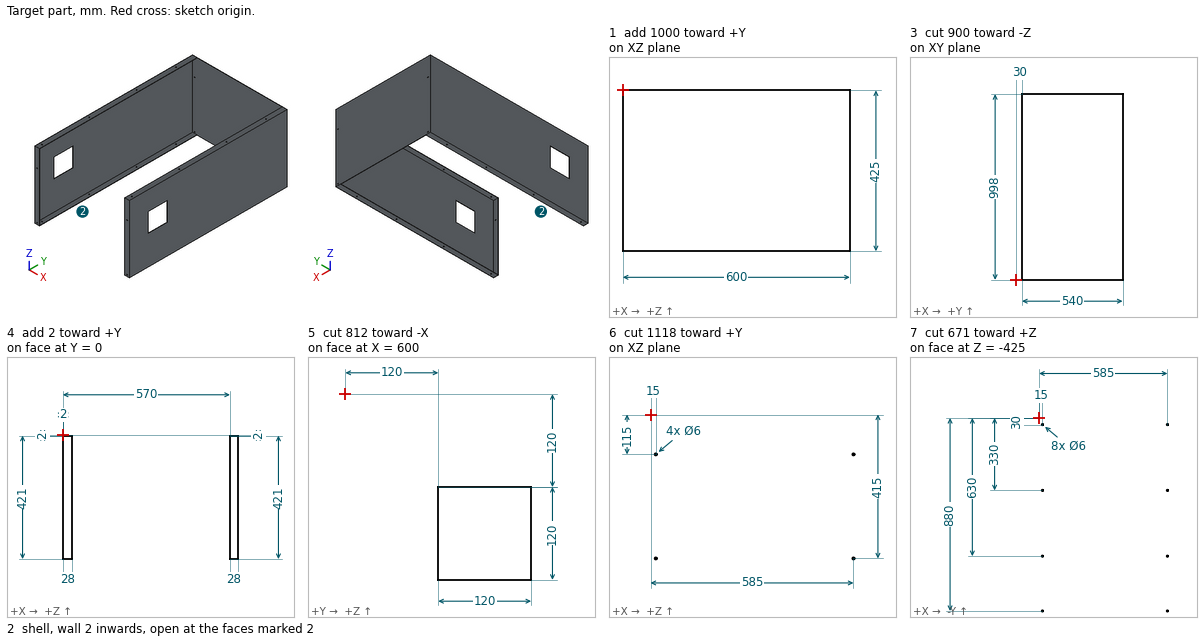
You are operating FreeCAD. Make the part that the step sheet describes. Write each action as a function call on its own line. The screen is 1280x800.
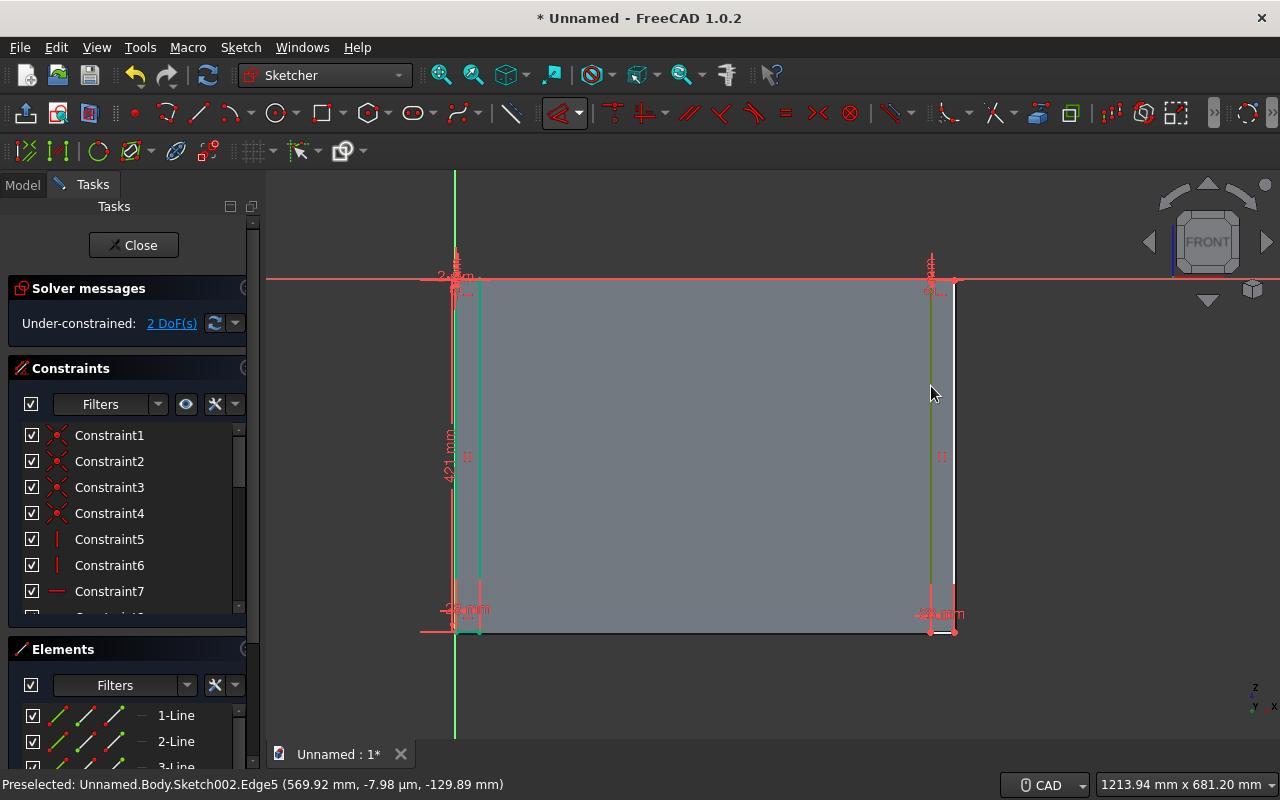
click(582, 114)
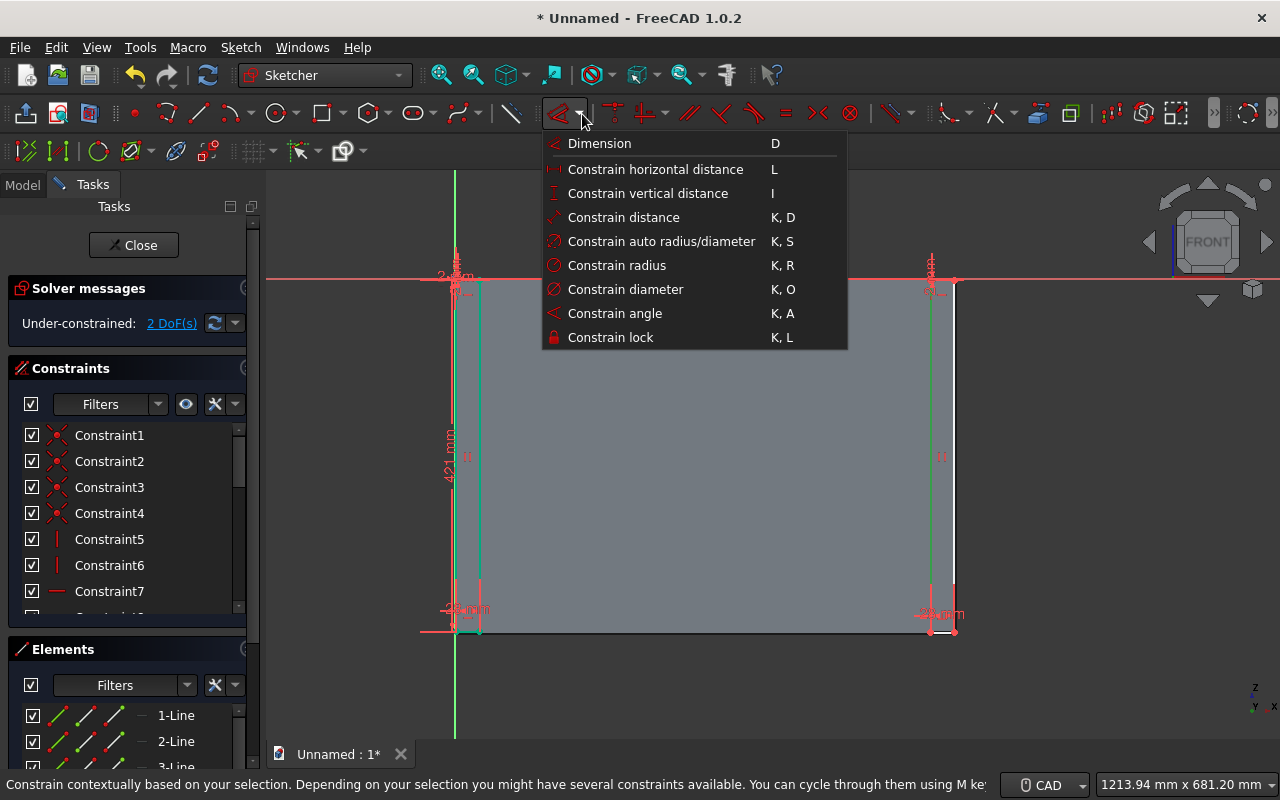
click(695, 193)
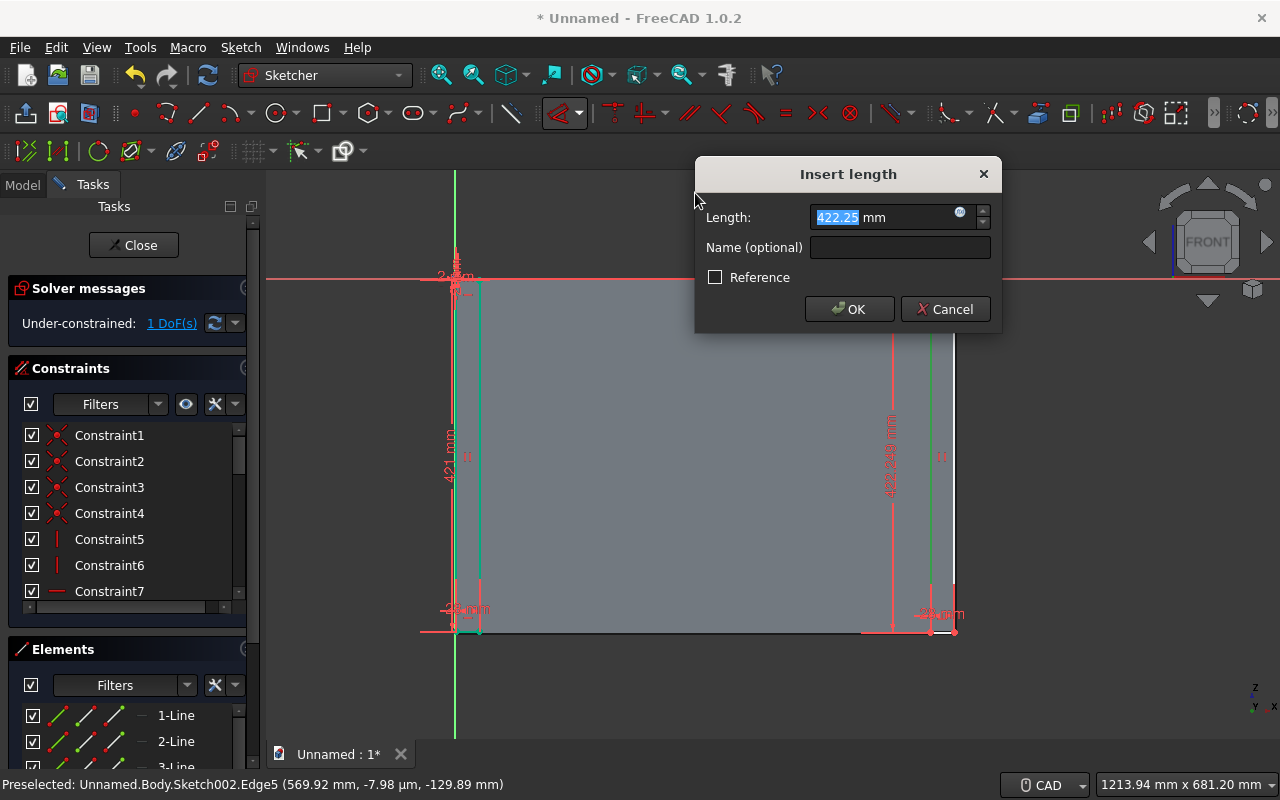
text(421)
key(Return)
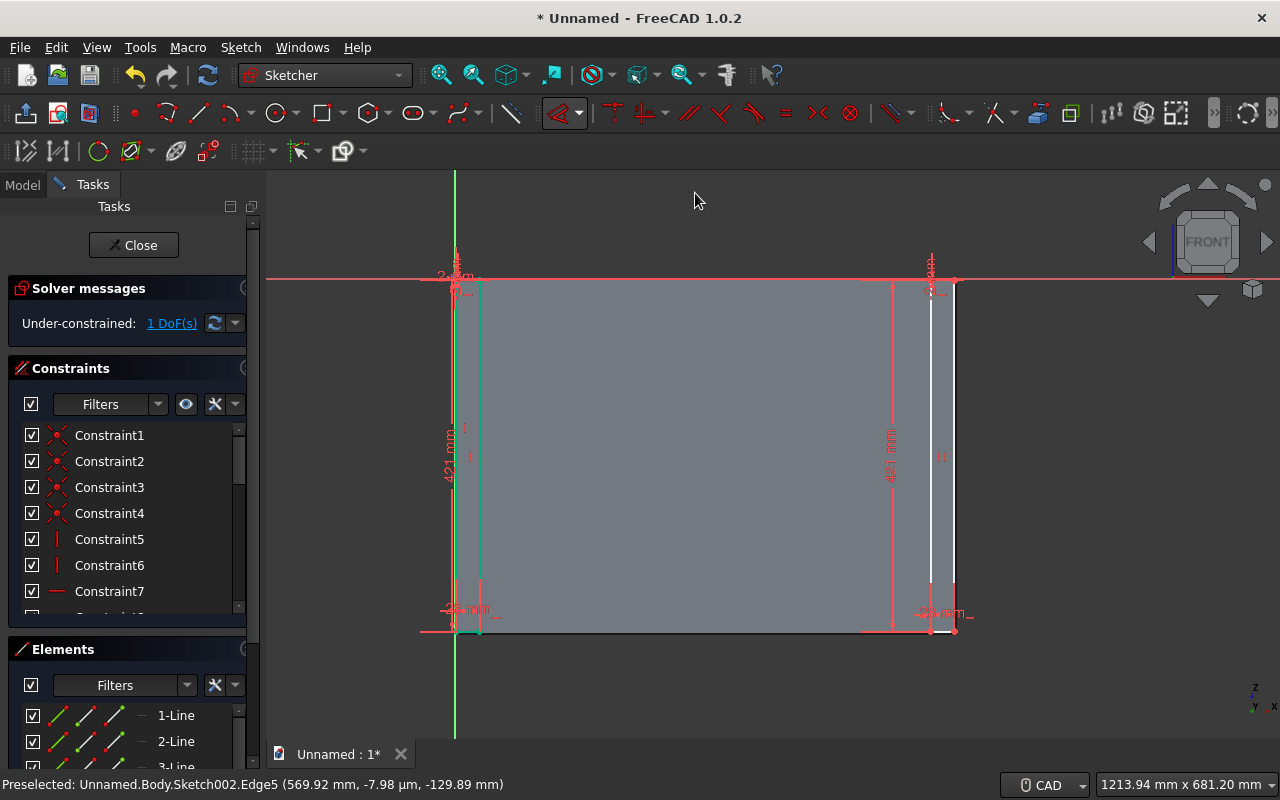
click(931, 280)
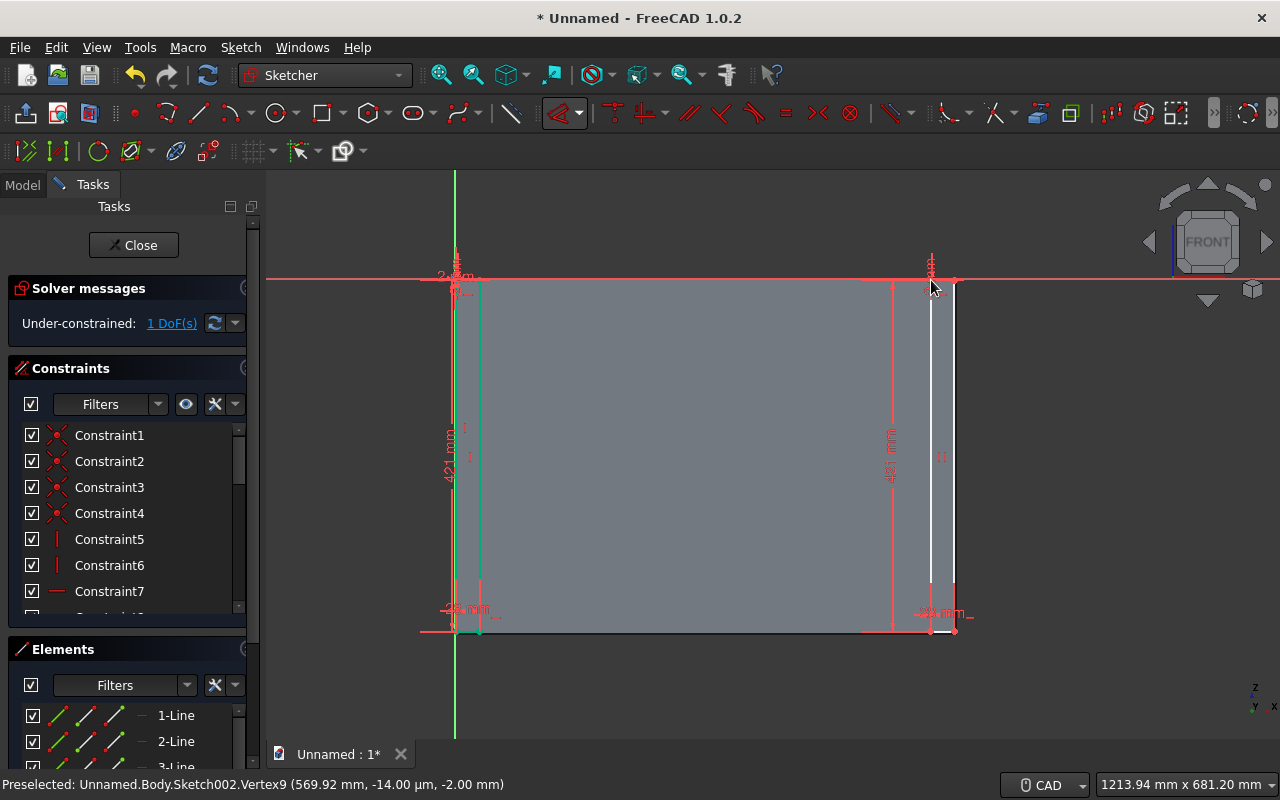
click(582, 114)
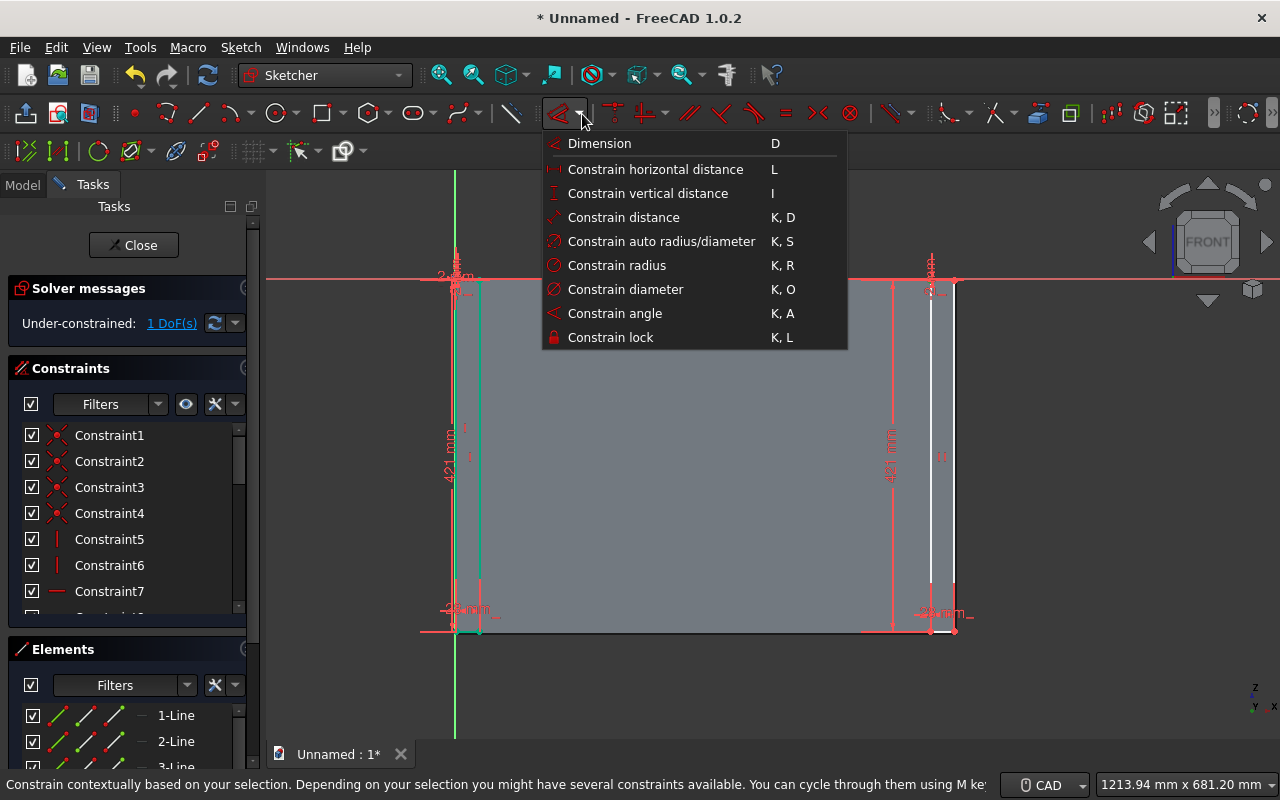
click(695, 169)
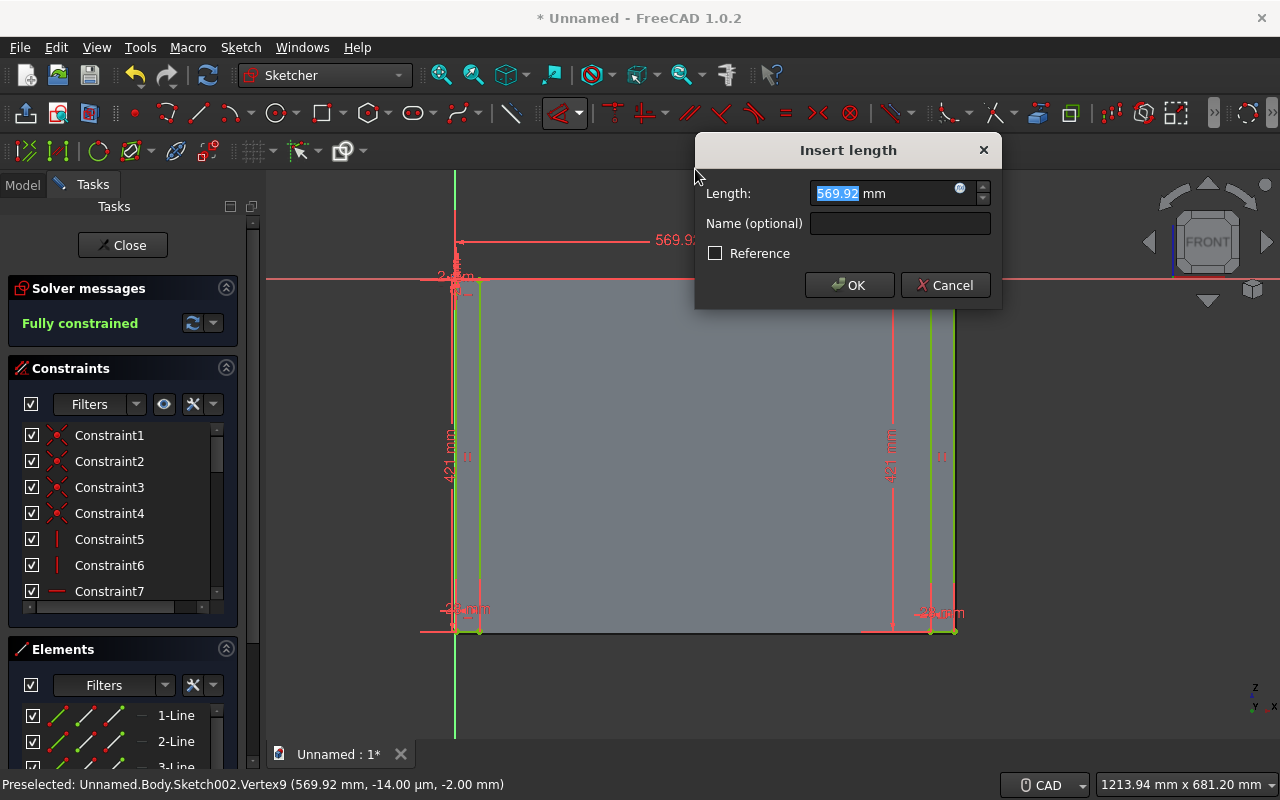
text(570)
key(Return)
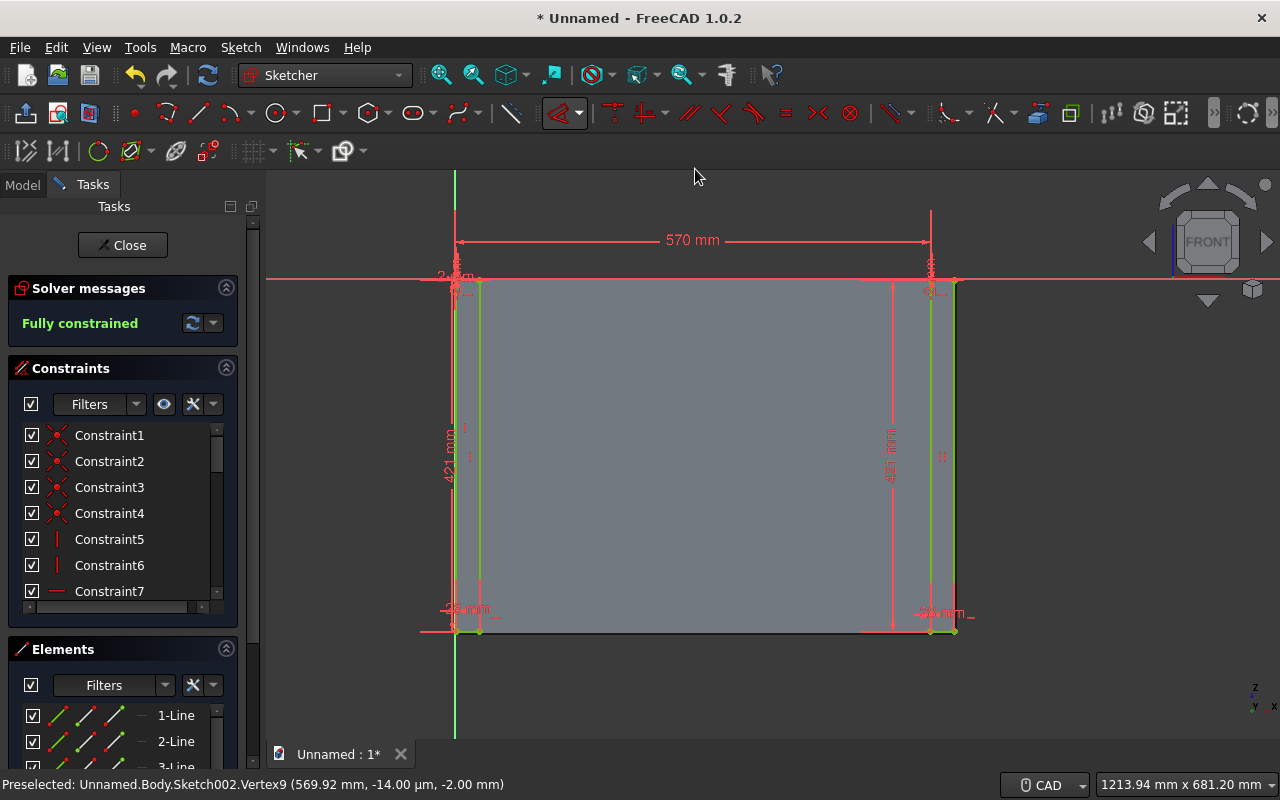
click(123, 245)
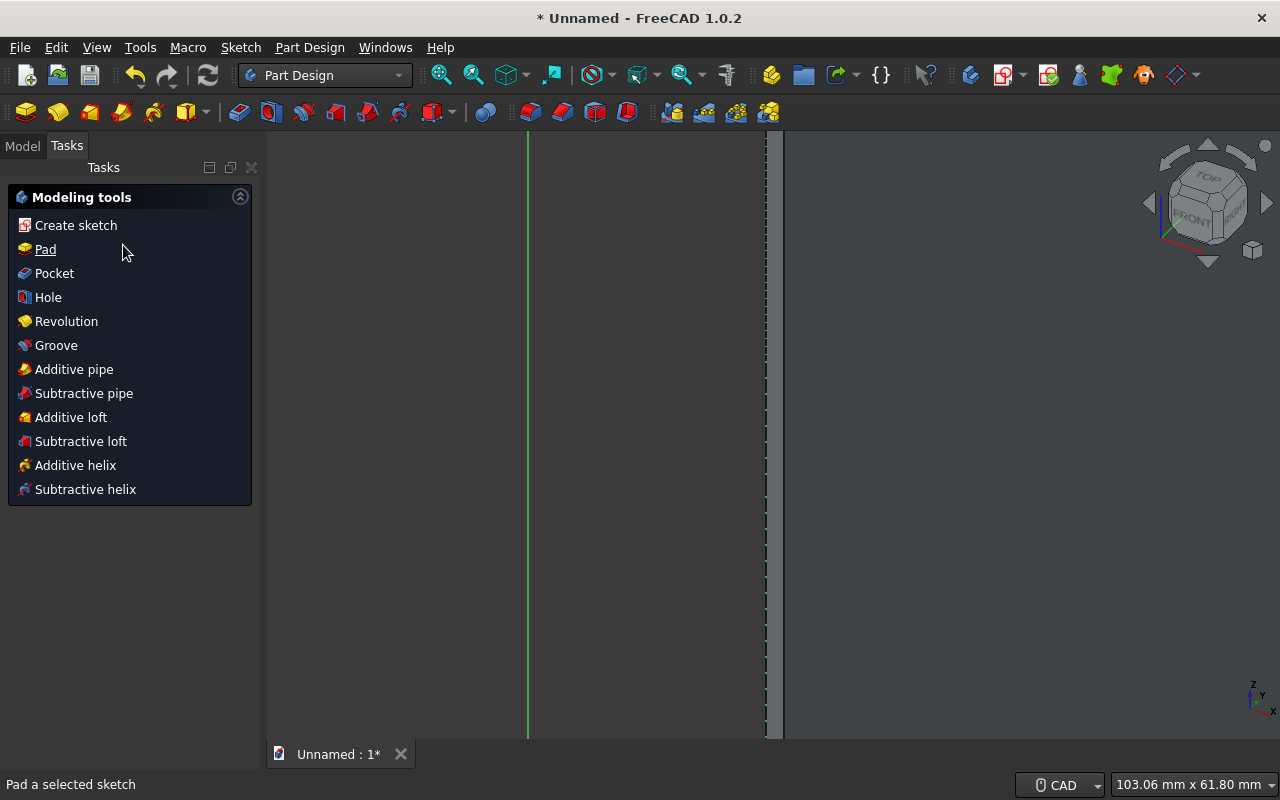
click(26, 112)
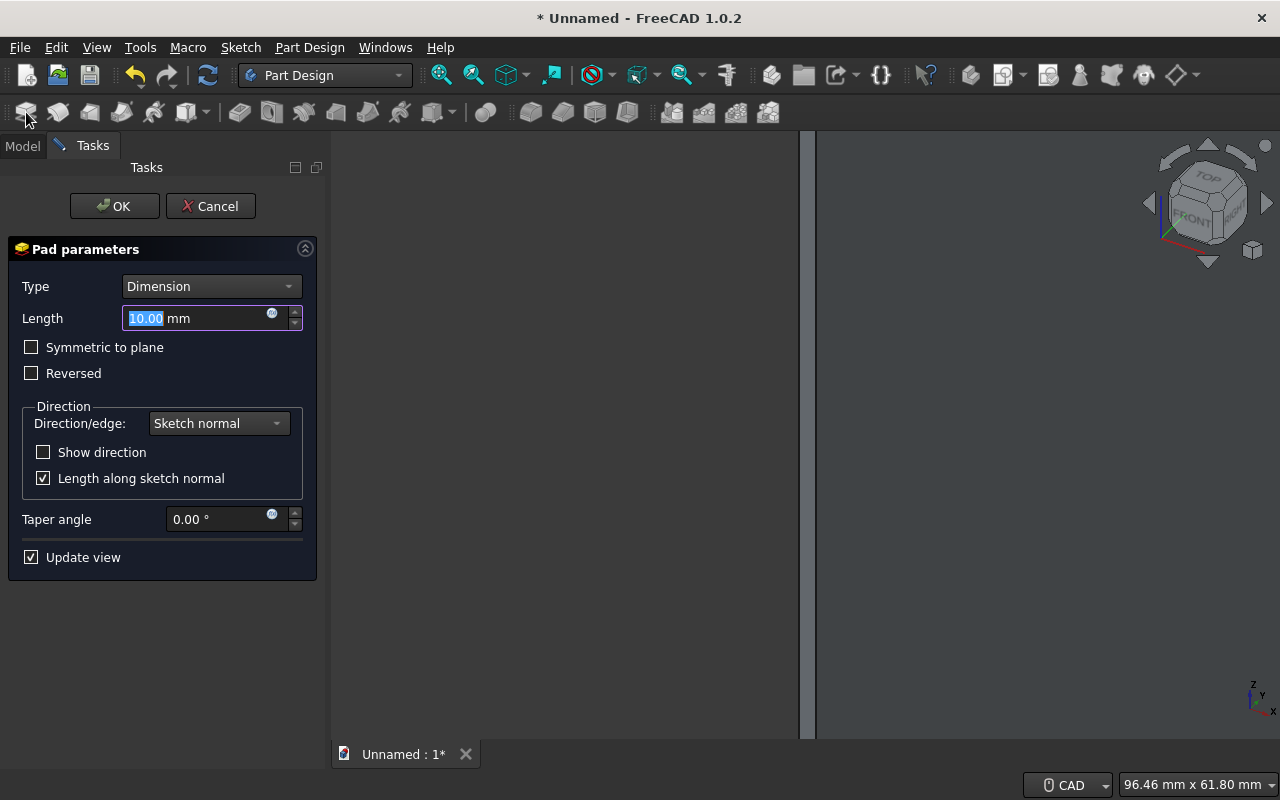
text(2)
key(Tab)